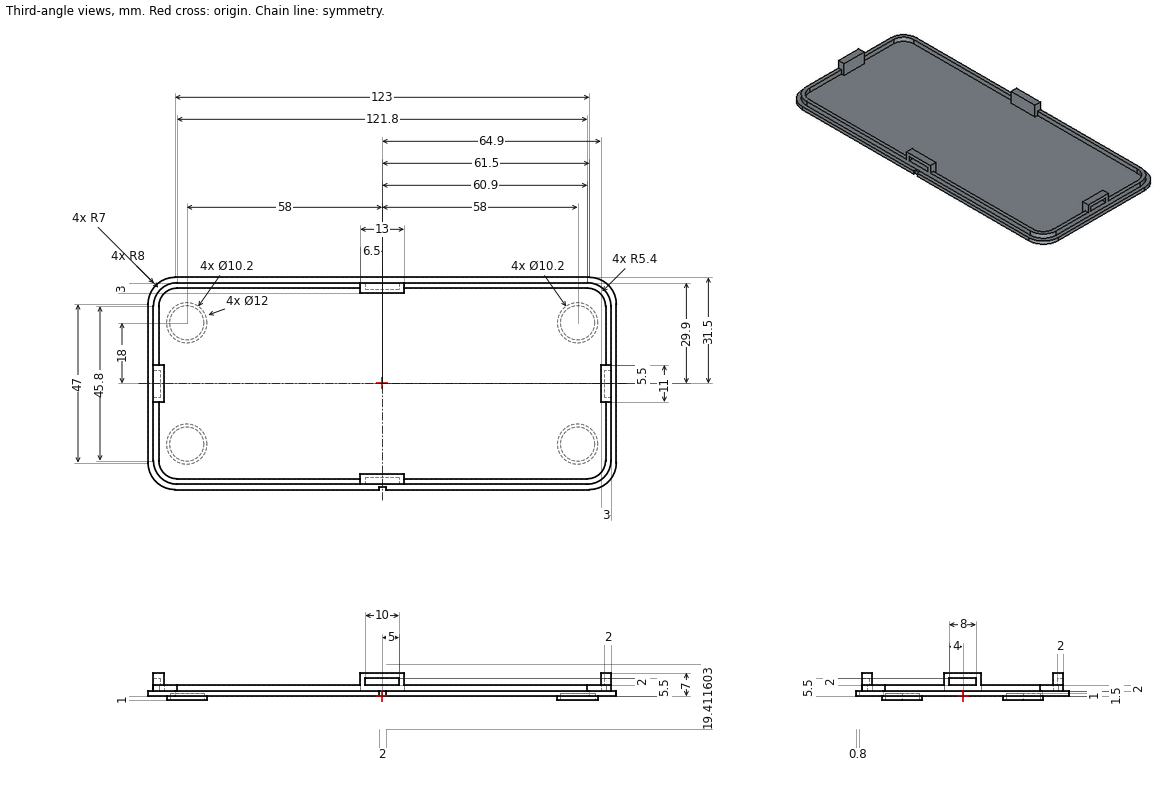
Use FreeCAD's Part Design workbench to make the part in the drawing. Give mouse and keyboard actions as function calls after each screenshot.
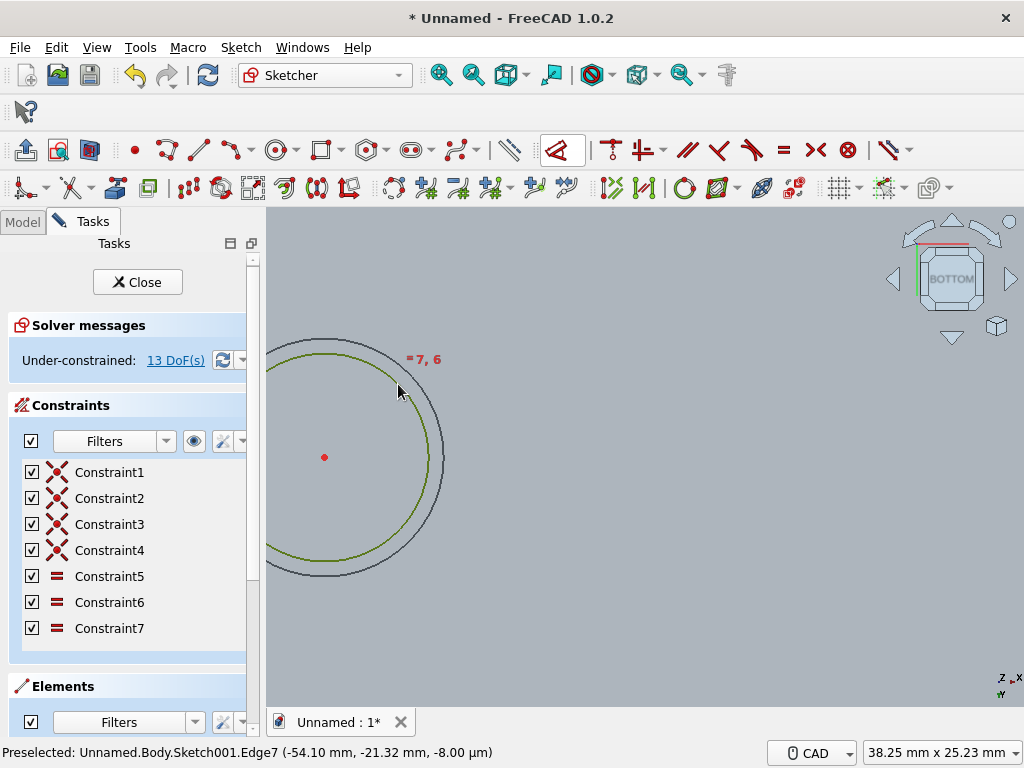
scroll(399, 387, down, 9)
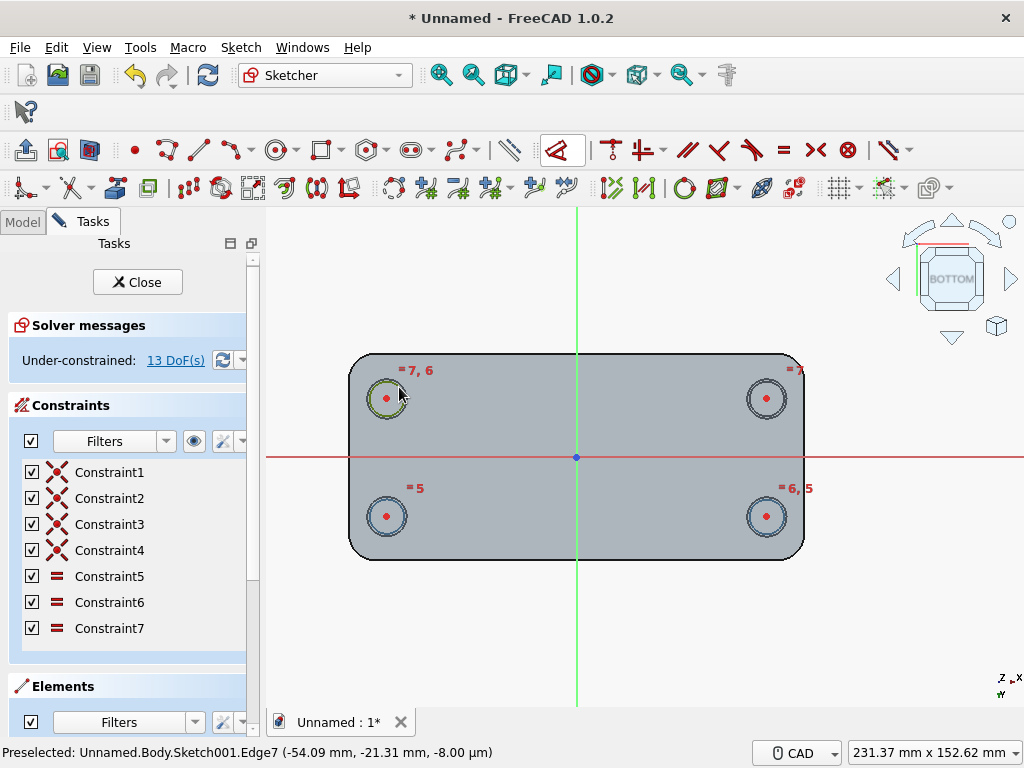
scroll(779, 387, up, 9)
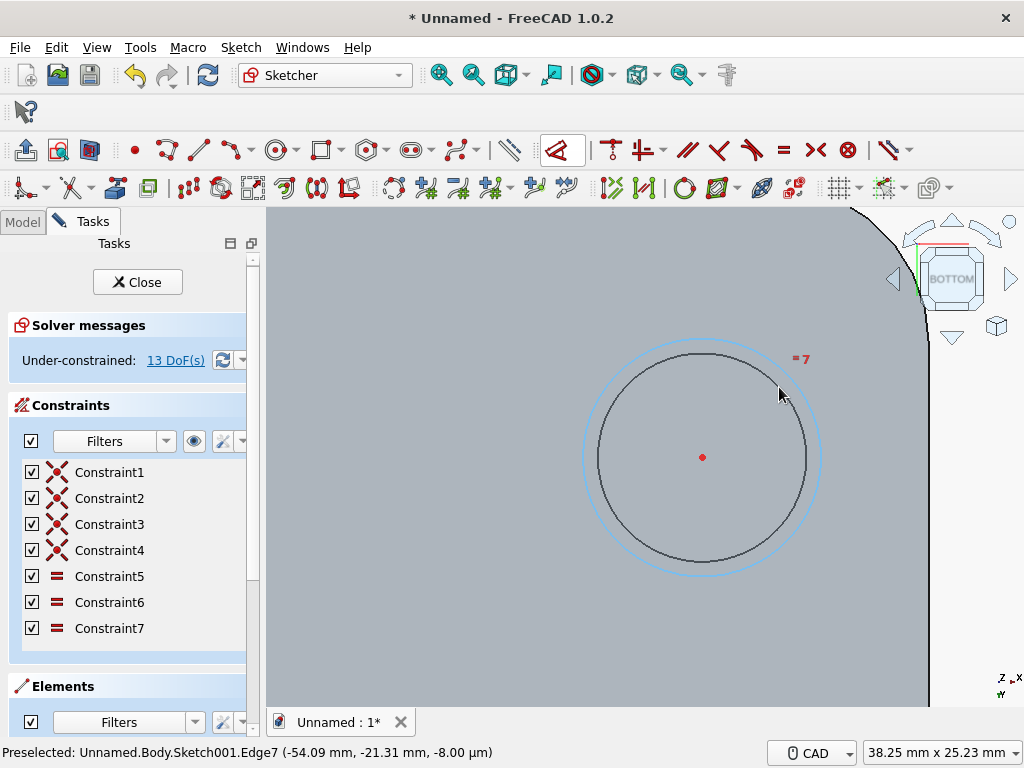
click(776, 384)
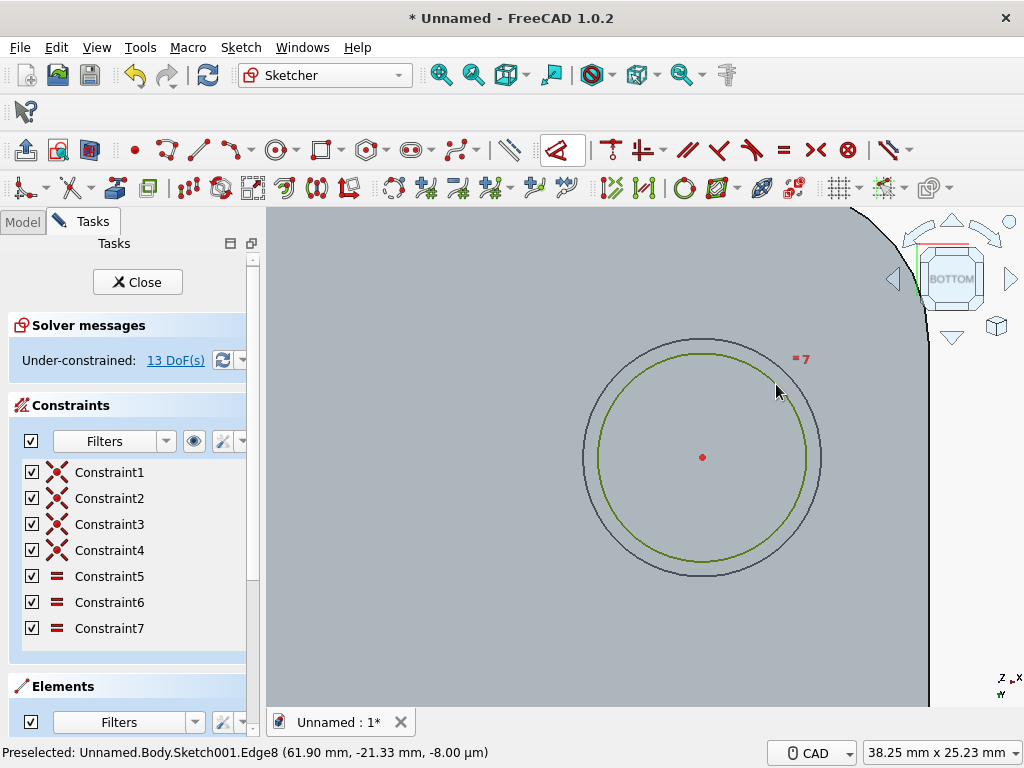
key(e)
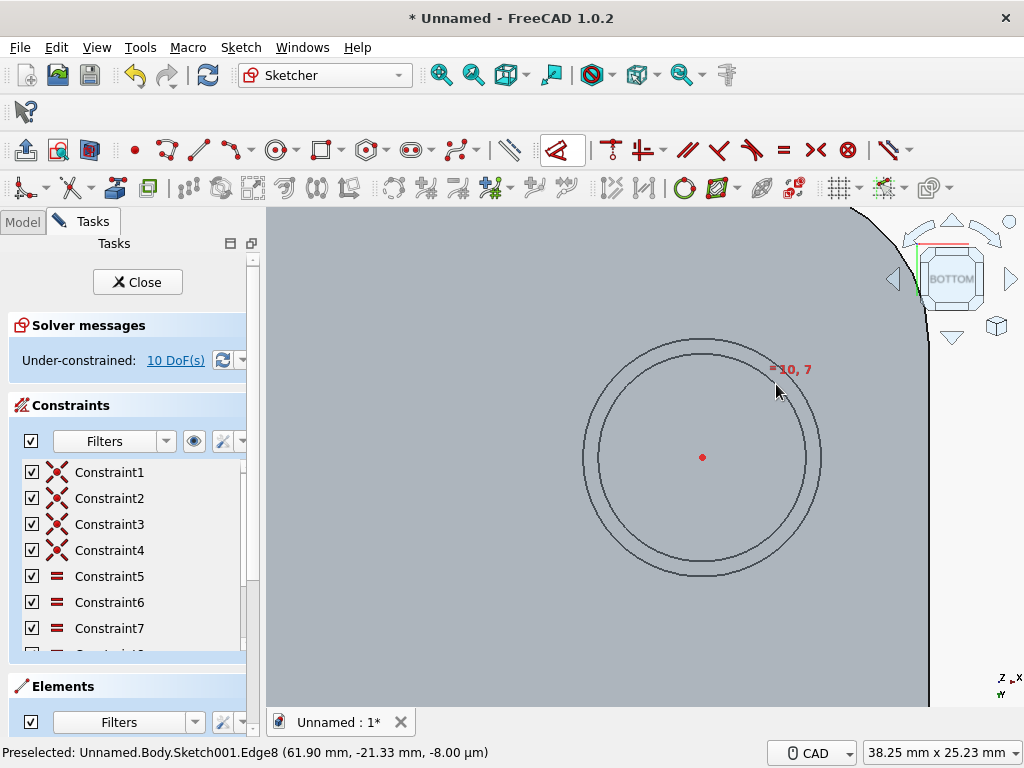
scroll(780, 387, down, 9)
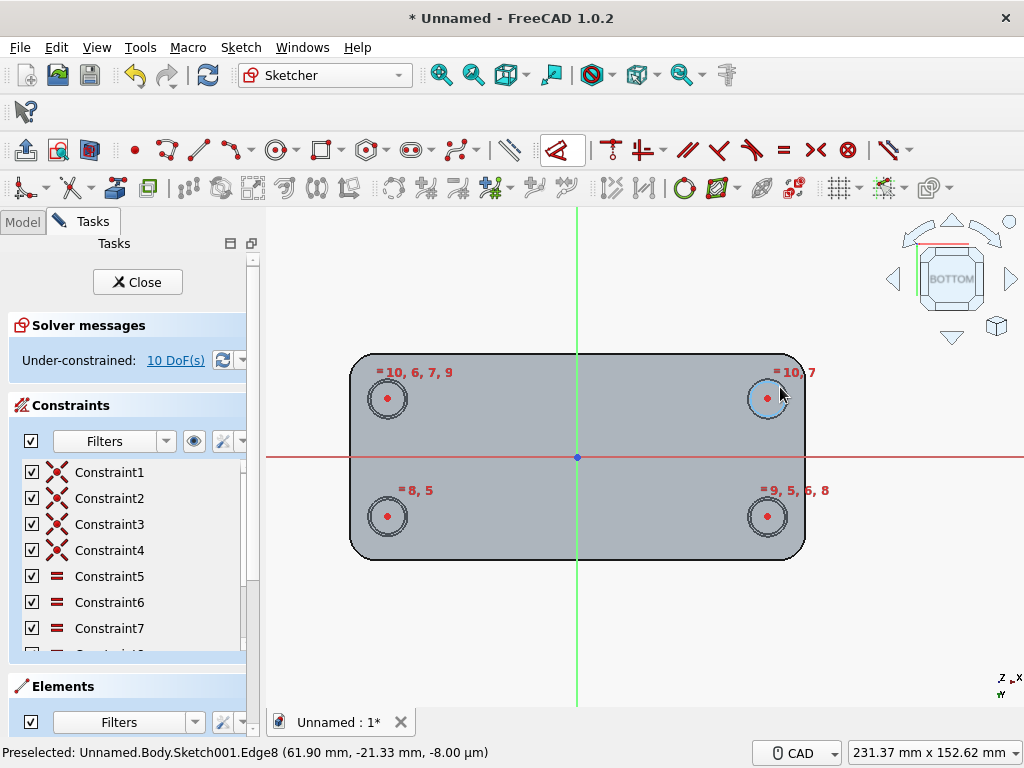
click(388, 517)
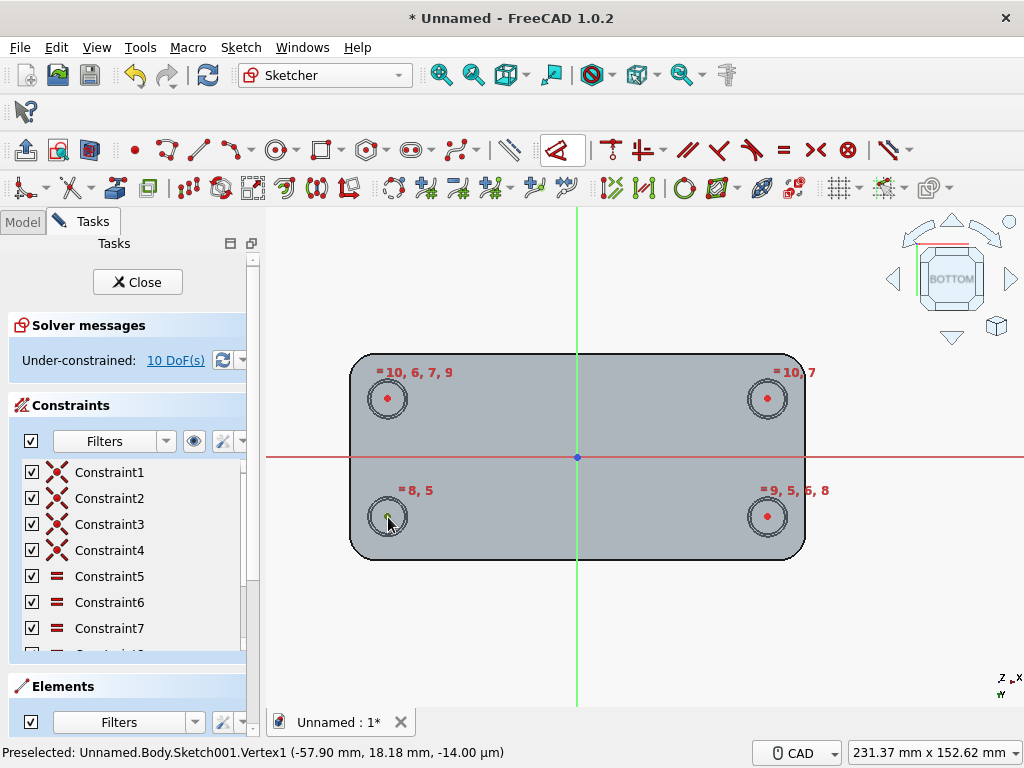
click(768, 517)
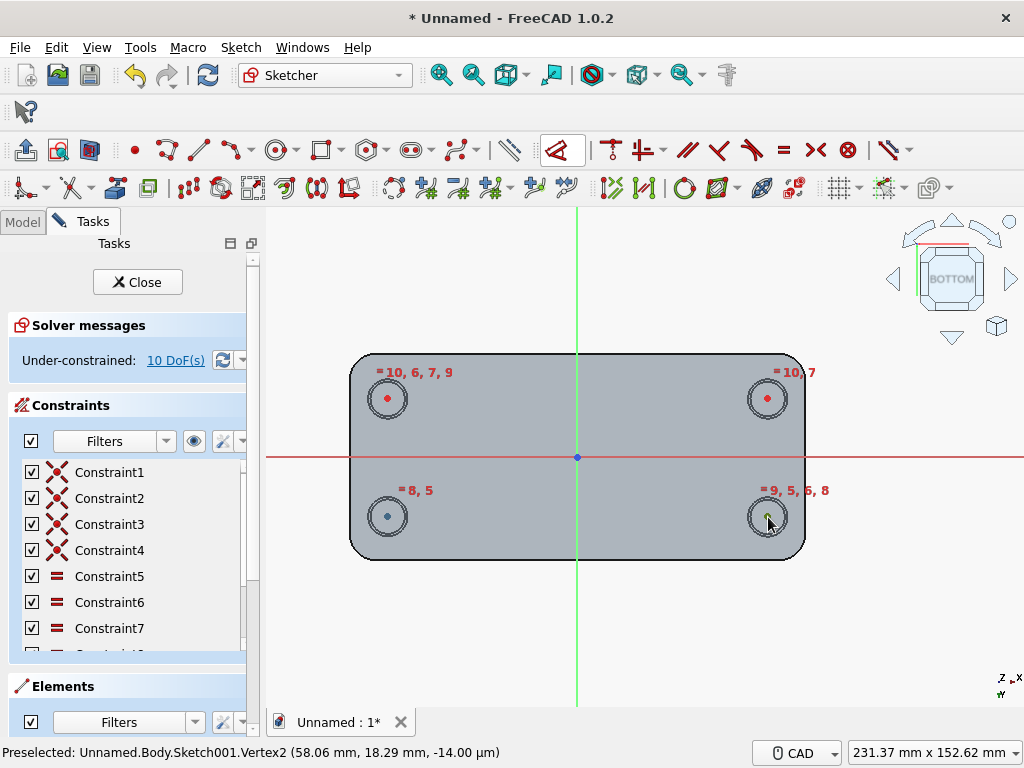
click(577, 647)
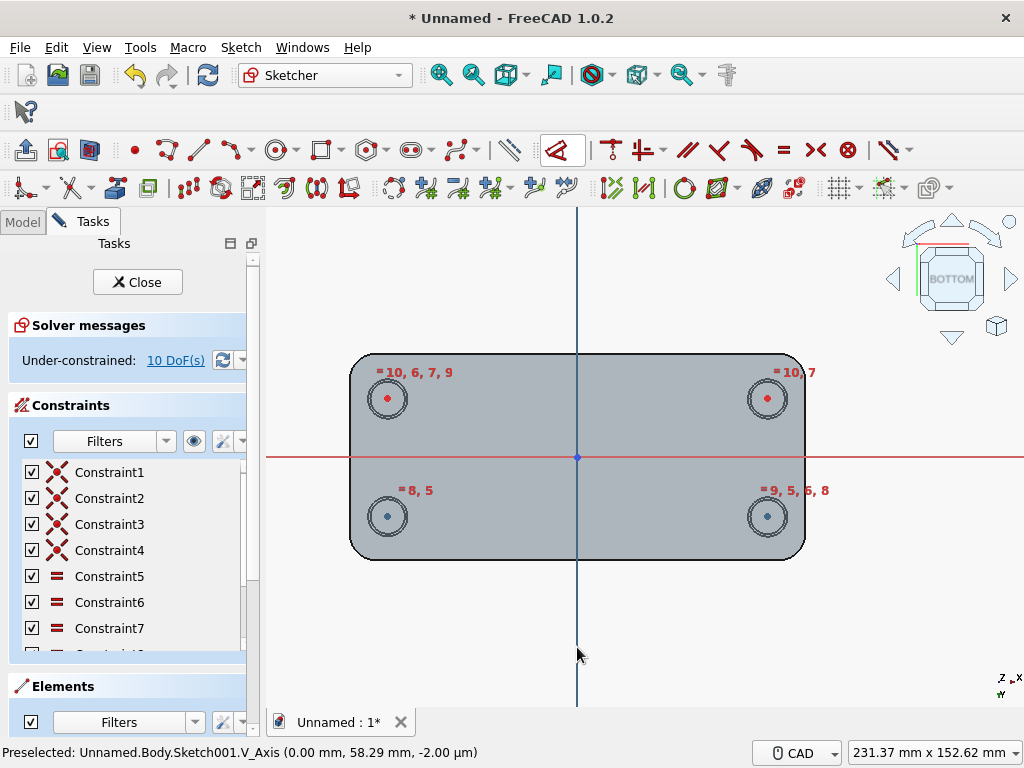
key(s)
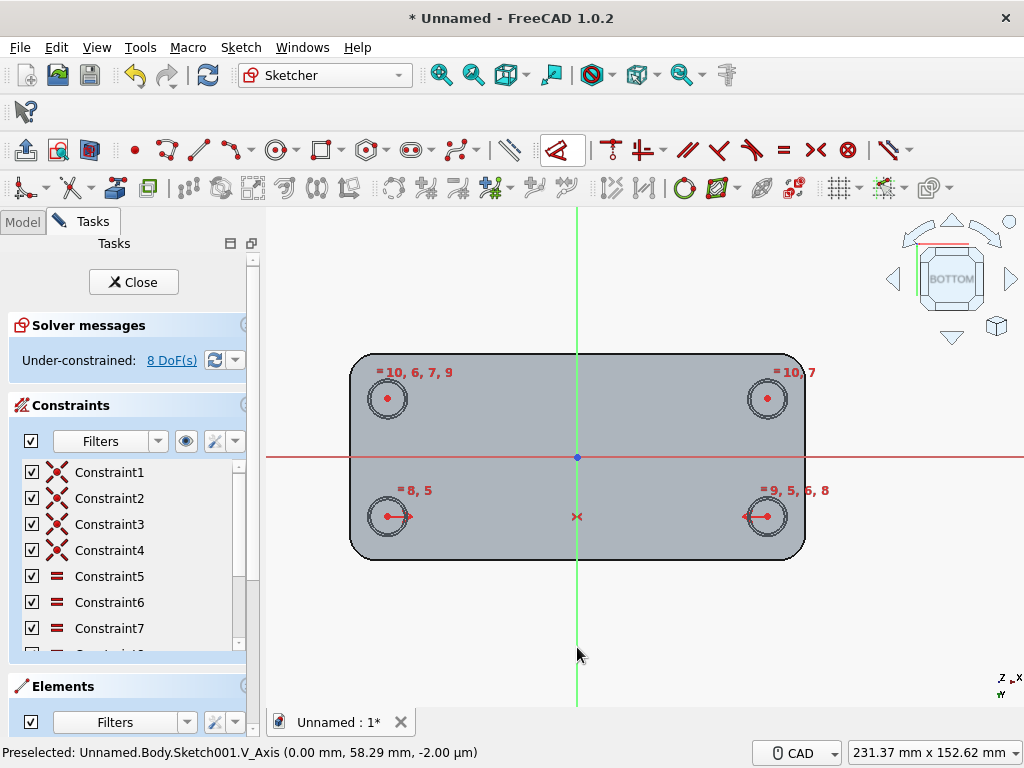
click(388, 517)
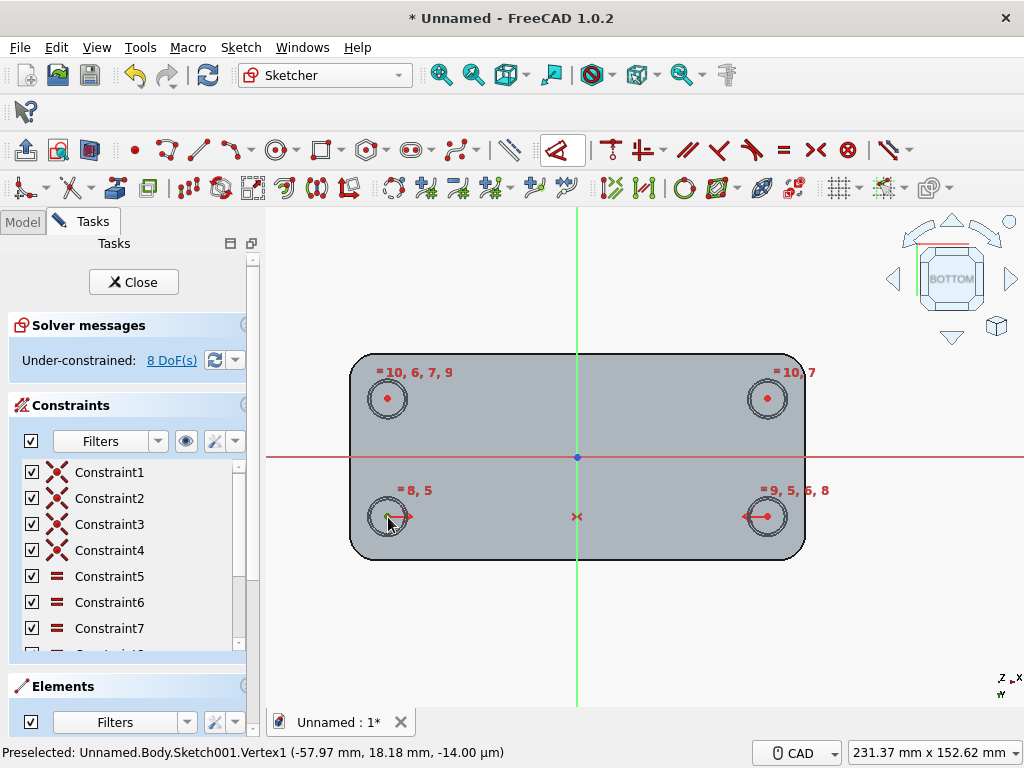
click(388, 399)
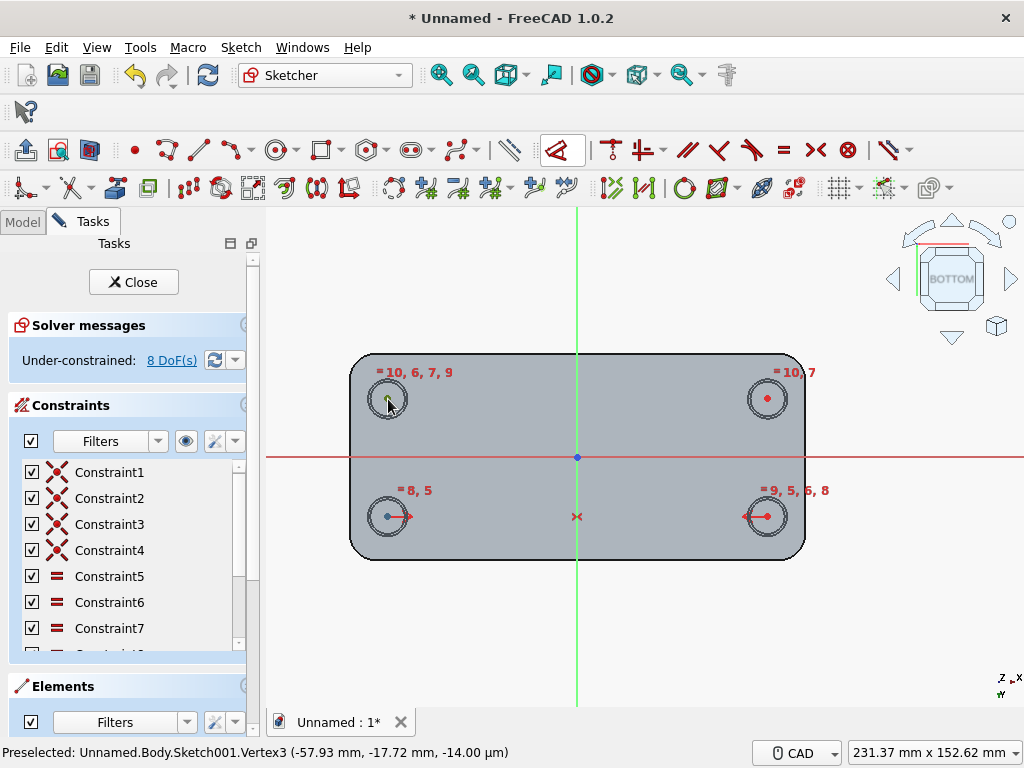
click(334, 457)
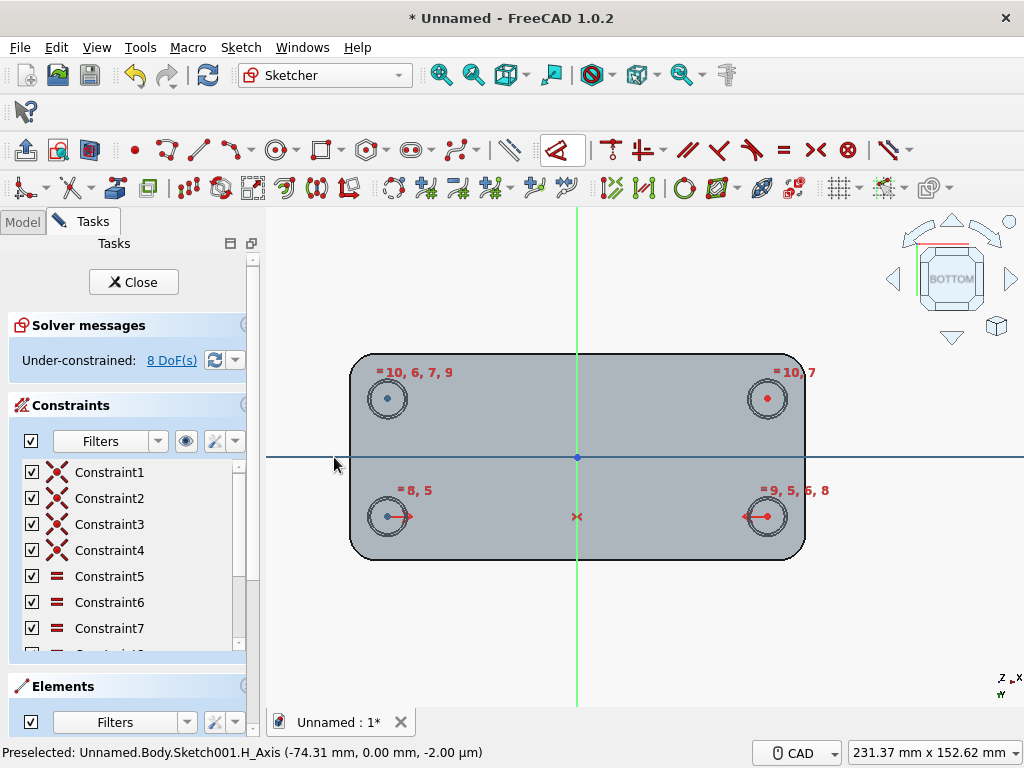
key(s)